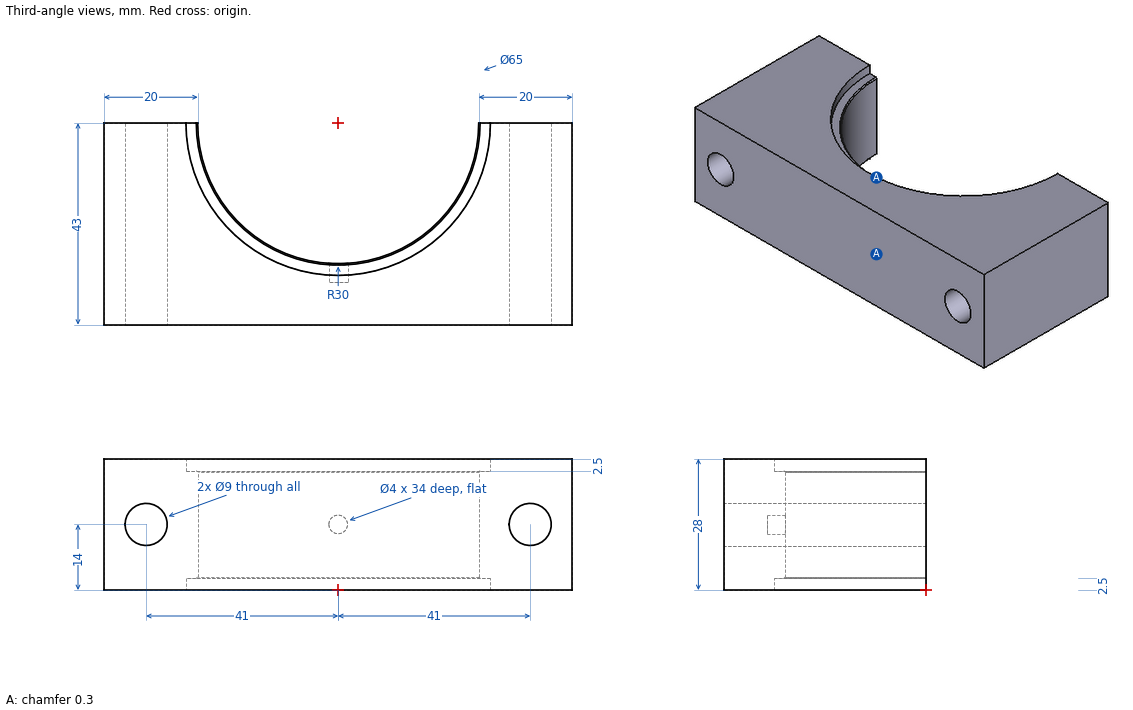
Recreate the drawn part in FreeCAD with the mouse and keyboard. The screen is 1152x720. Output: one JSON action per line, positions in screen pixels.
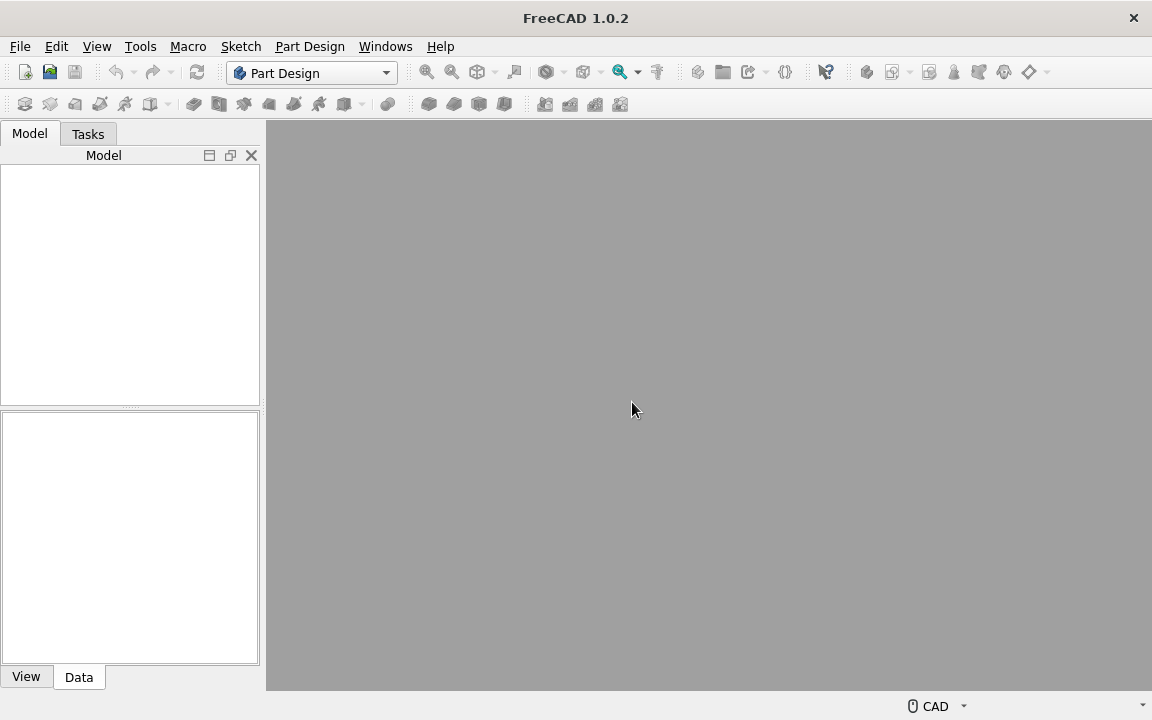
{"action": "left_click", "coordinate": [25, 72]}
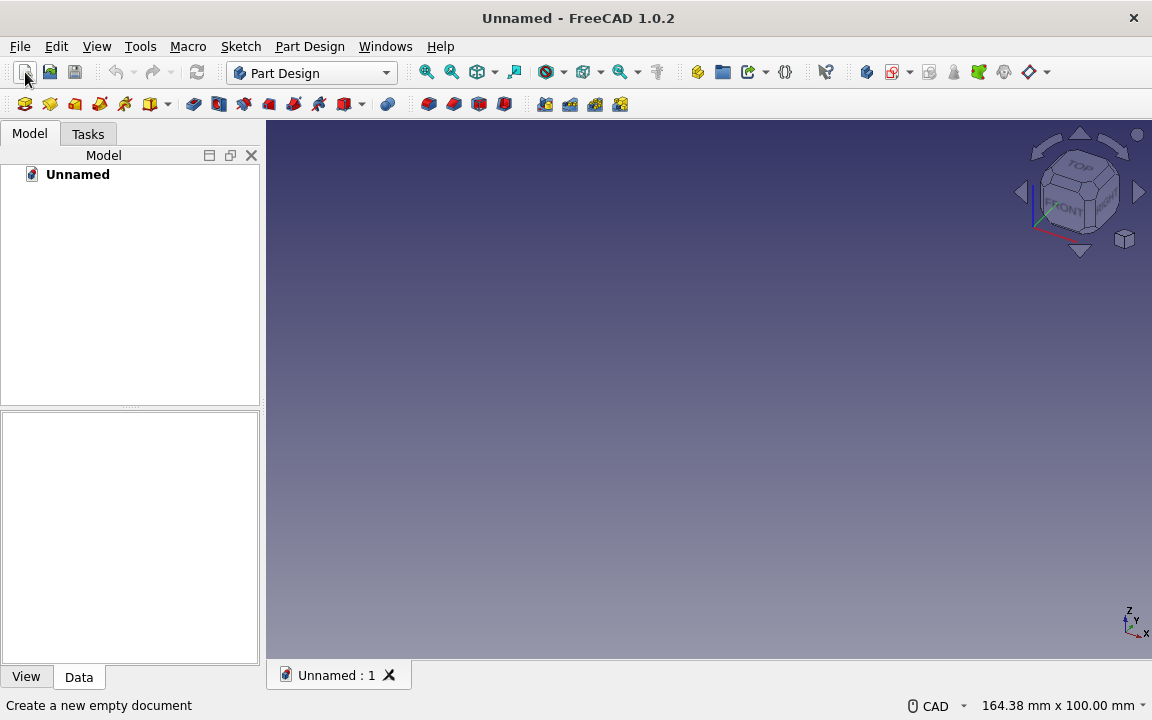
{"action": "left_click", "coordinate": [892, 72]}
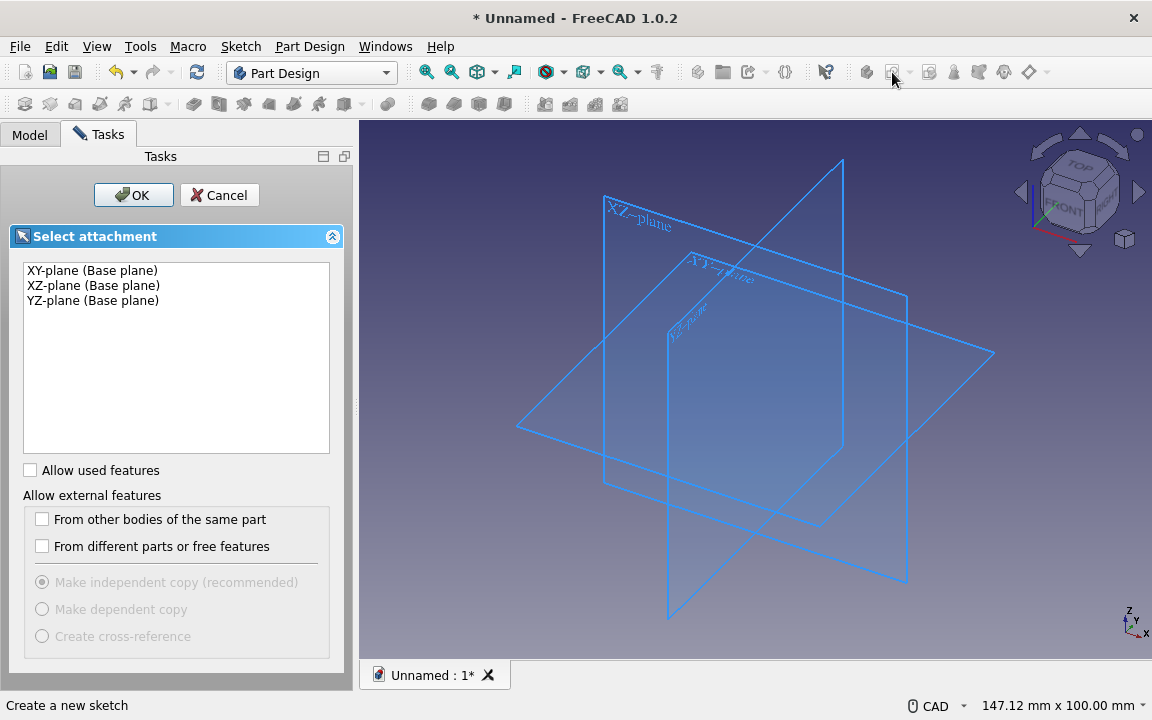
{"action": "left_click", "coordinate": [84, 270]}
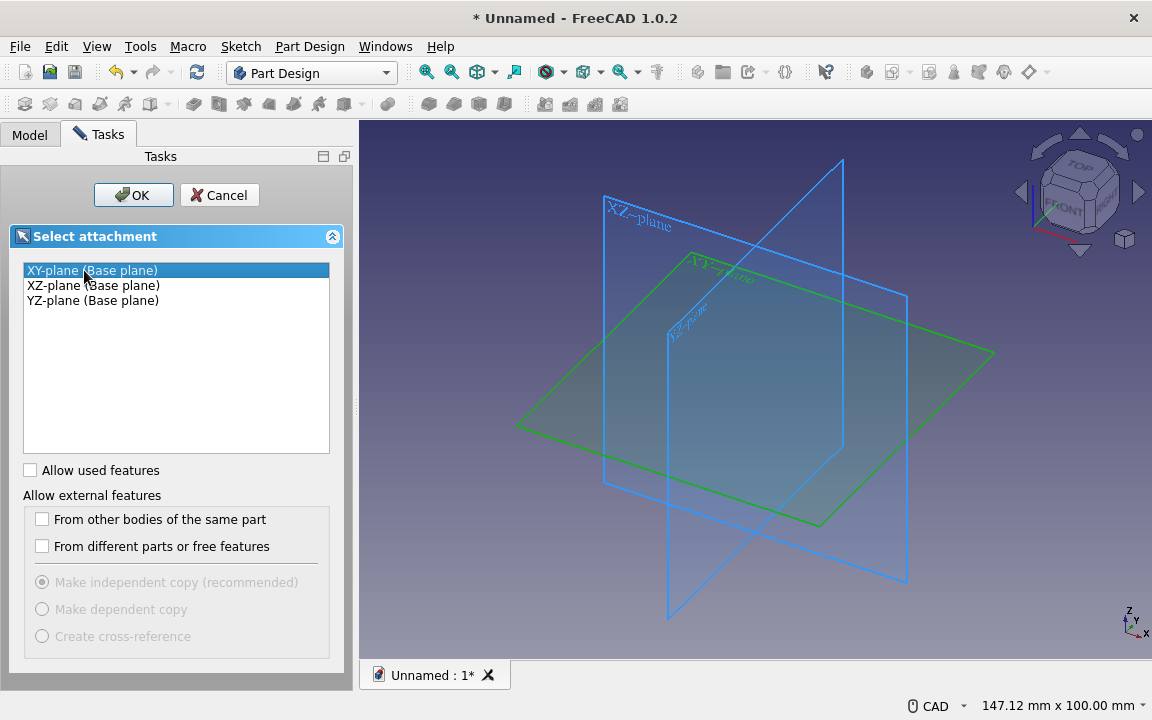
{"action": "left_click", "coordinate": [134, 195]}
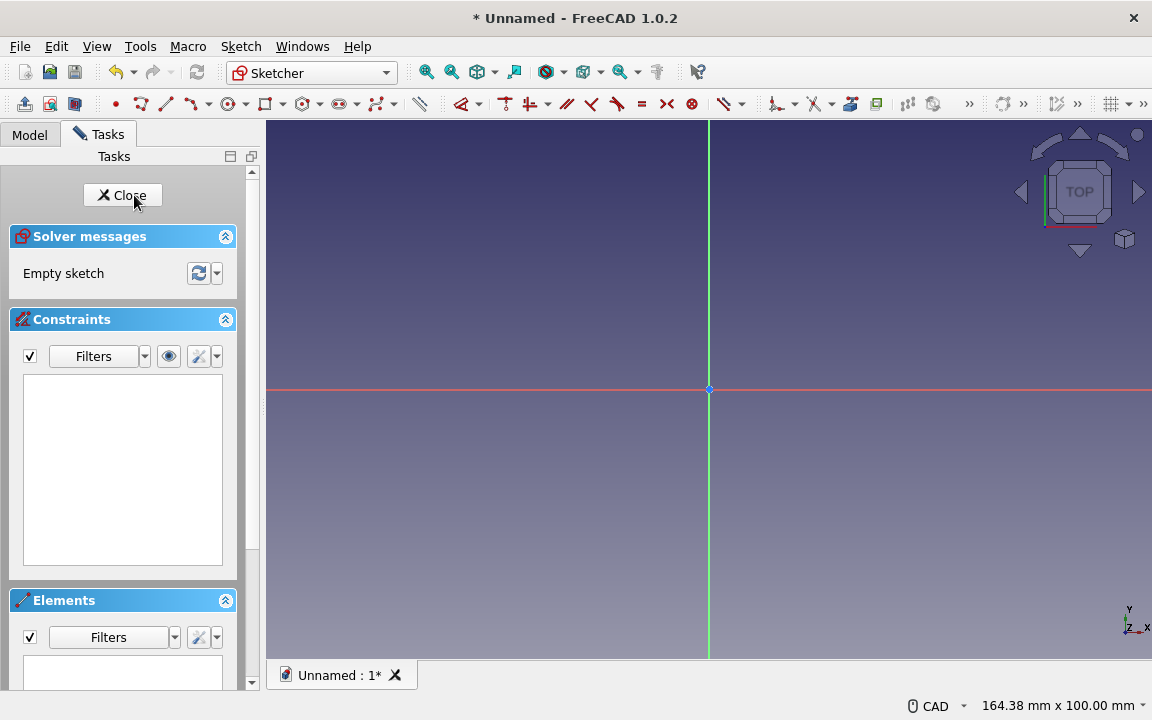
{"action": "scroll", "coordinate": [331, 148], "scroll_direction": "down", "scroll_amount": 1}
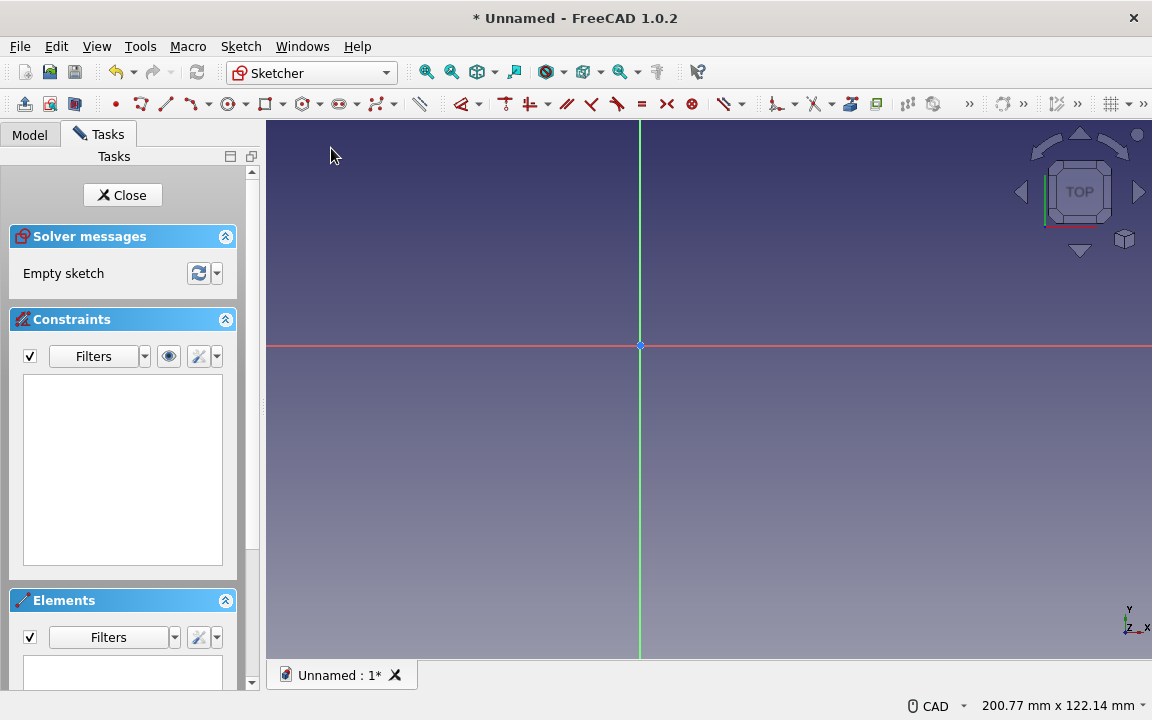
{"action": "left_click", "coordinate": [141, 104]}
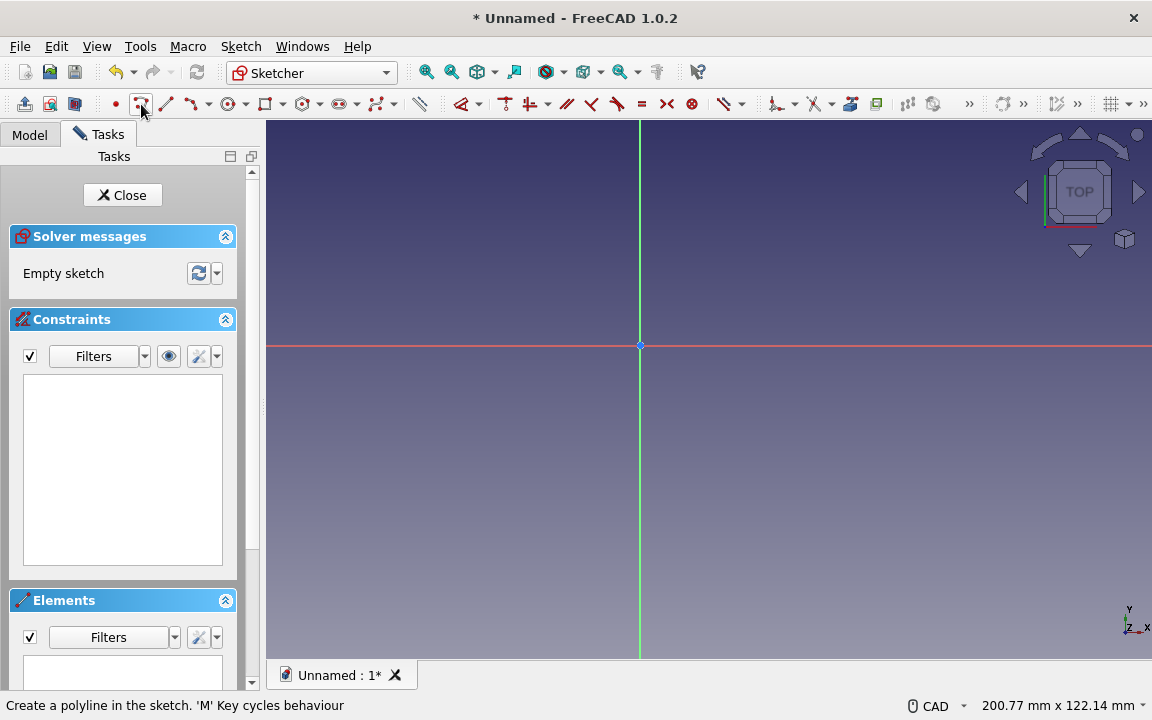
{"action": "left_click", "coordinate": [508, 346]}
{"action": "left_click", "coordinate": [420, 355]}
{"action": "left_click", "coordinate": [420, 535]}
{"action": "left_click", "coordinate": [861, 535]}
{"action": "left_click", "coordinate": [861, 346]}
{"action": "left_click", "coordinate": [773, 355]}
{"action": "right_click", "coordinate": [773, 355]}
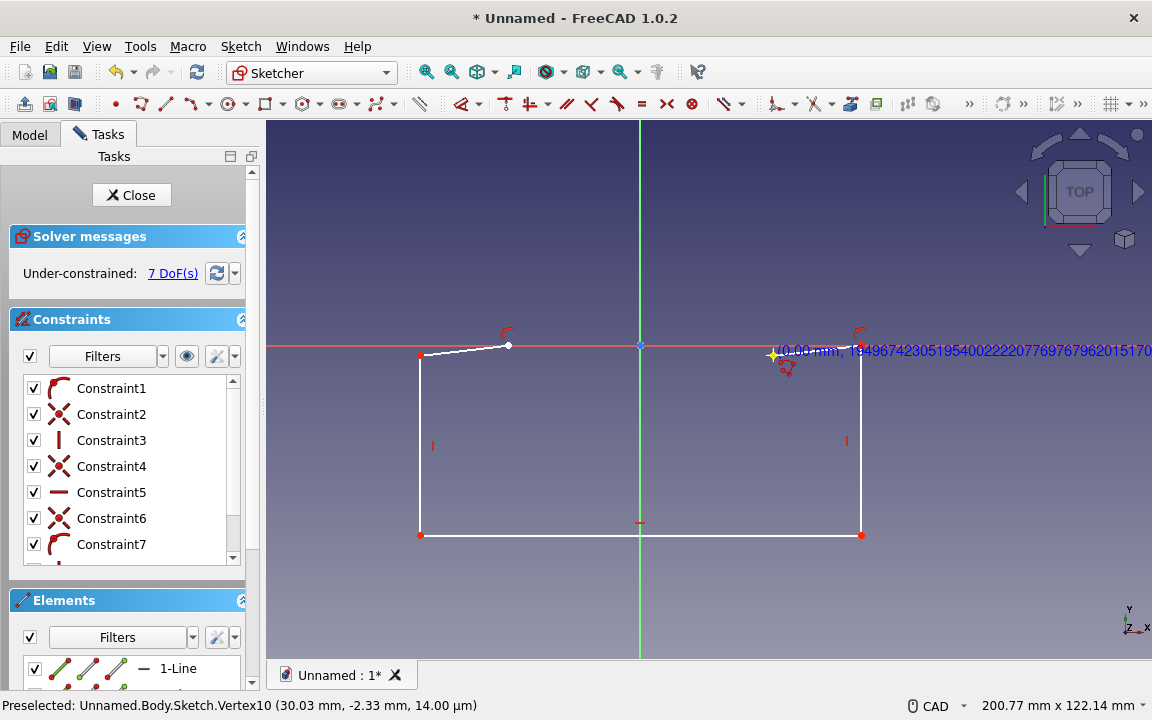
{"action": "left_click", "coordinate": [190, 104]}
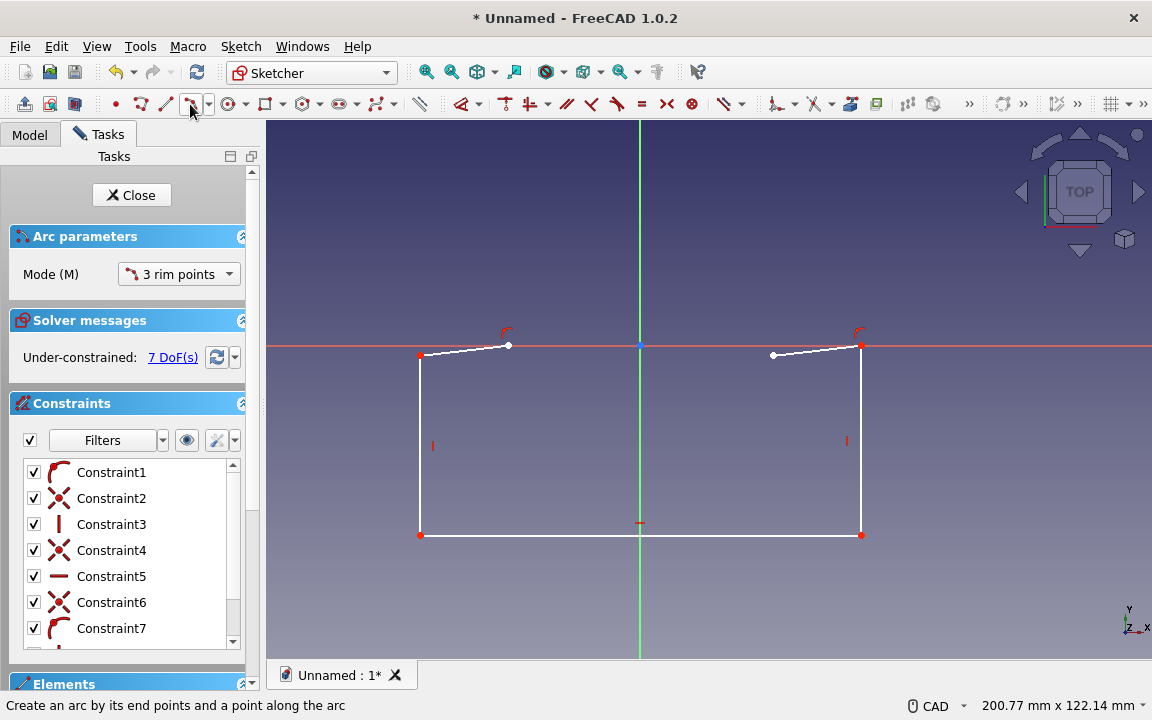
{"action": "left_click", "coordinate": [773, 356]}
{"action": "left_click", "coordinate": [508, 346]}
{"action": "left_click", "coordinate": [600, 472]}
{"action": "key", "text": "Escape"}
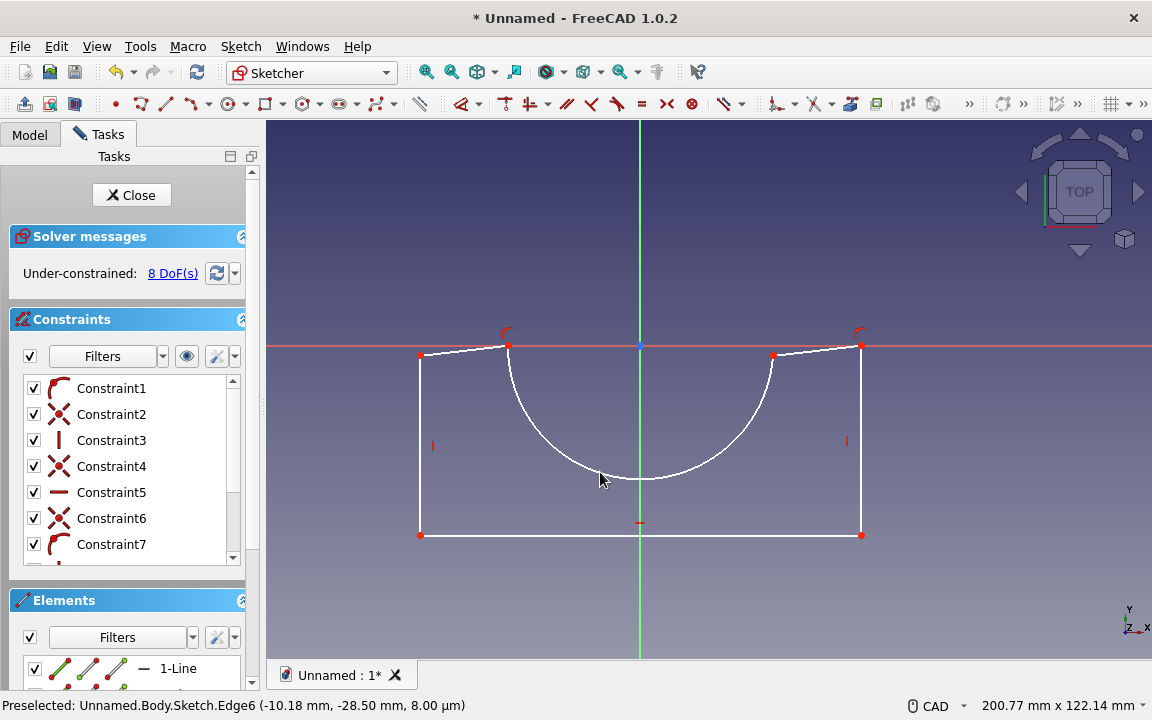
{"action": "left_click", "coordinate": [482, 349]}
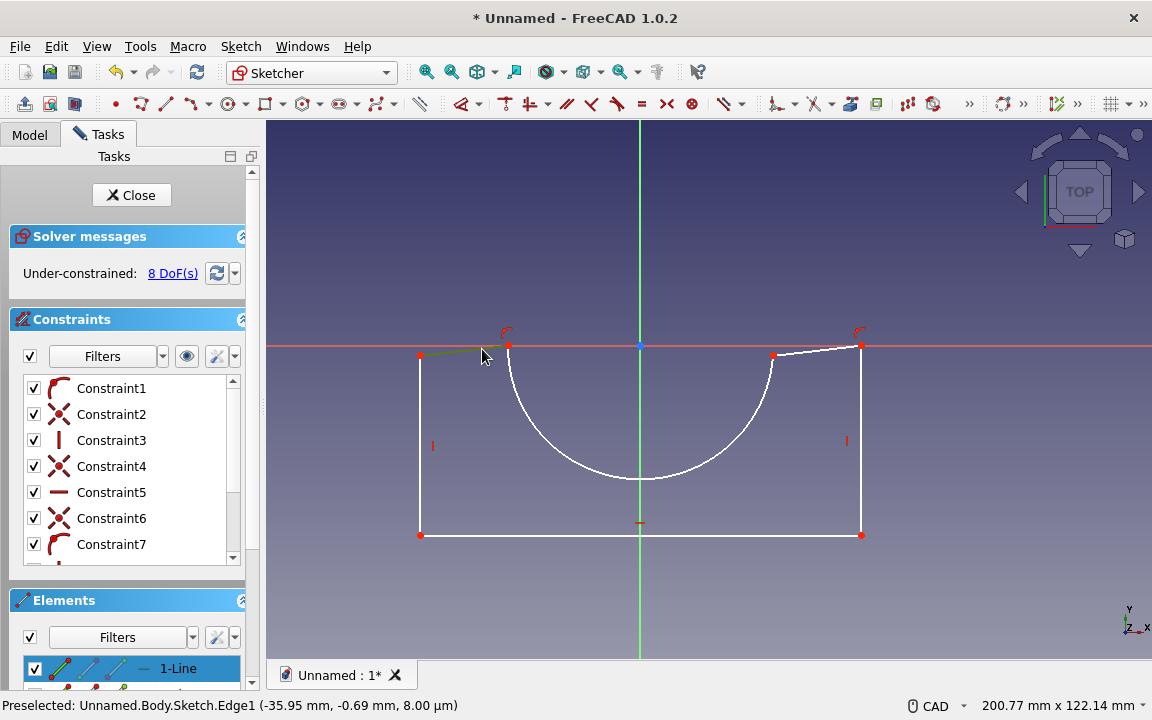
{"action": "left_click", "coordinate": [548, 104]}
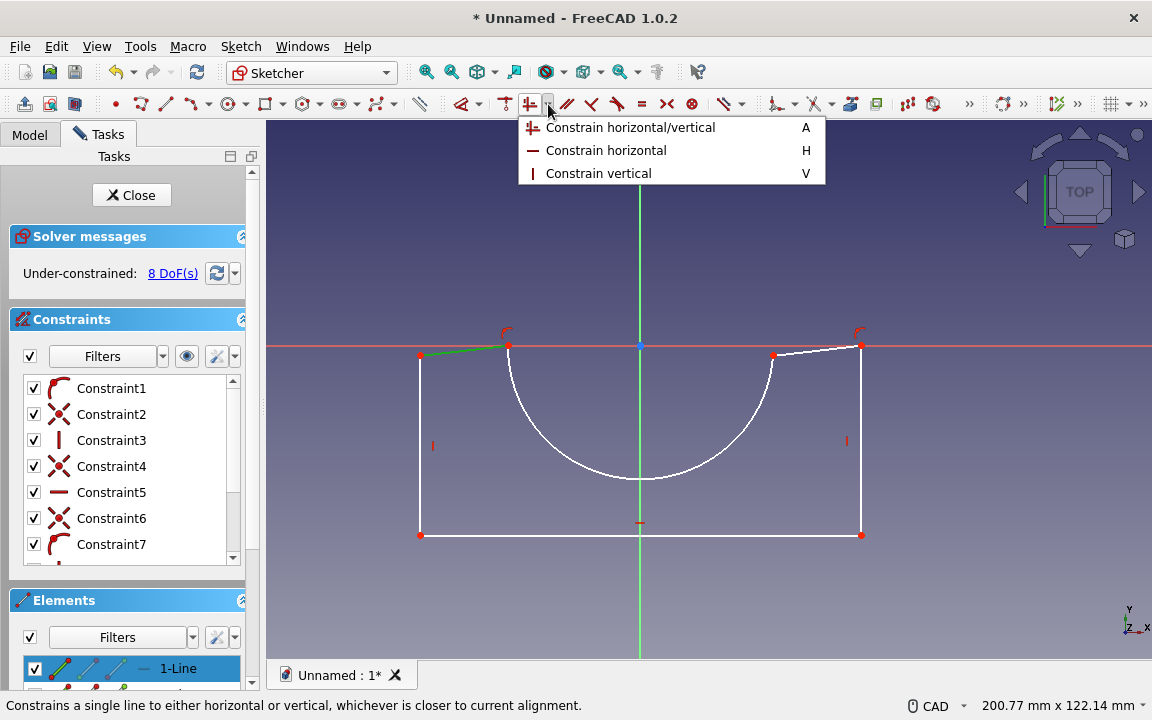
{"action": "left_click", "coordinate": [672, 150]}